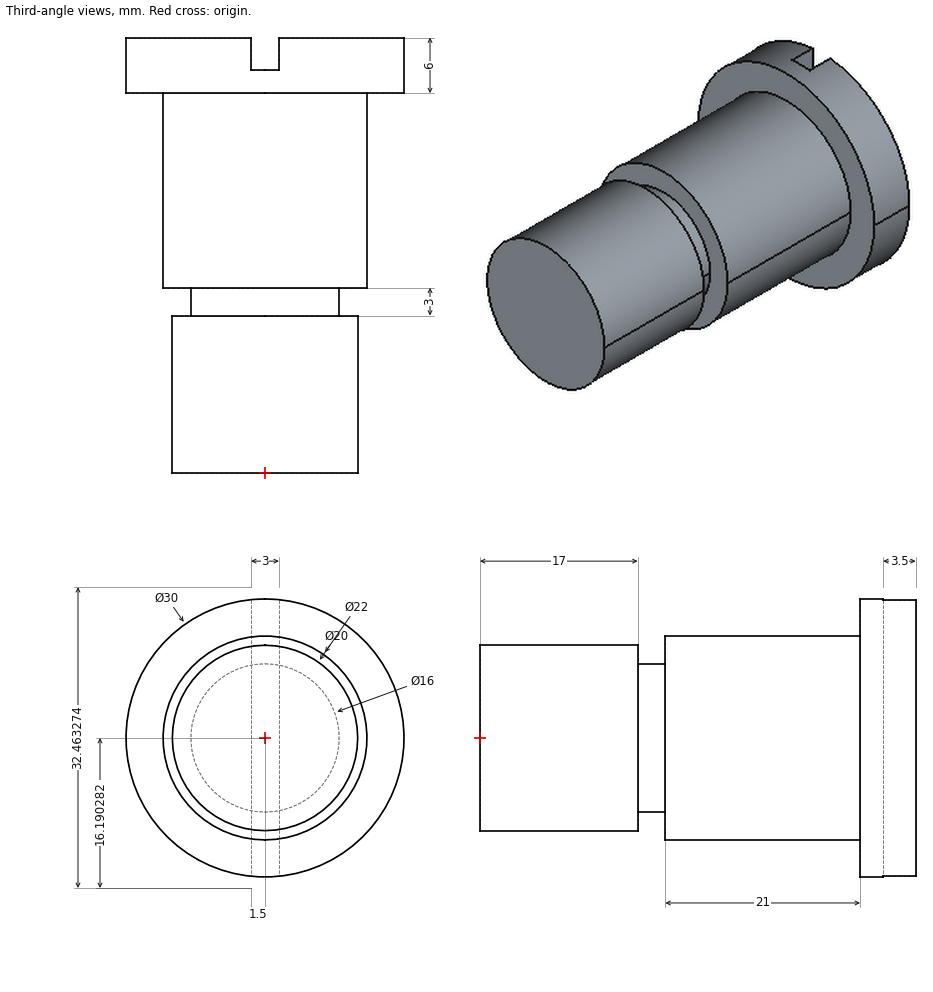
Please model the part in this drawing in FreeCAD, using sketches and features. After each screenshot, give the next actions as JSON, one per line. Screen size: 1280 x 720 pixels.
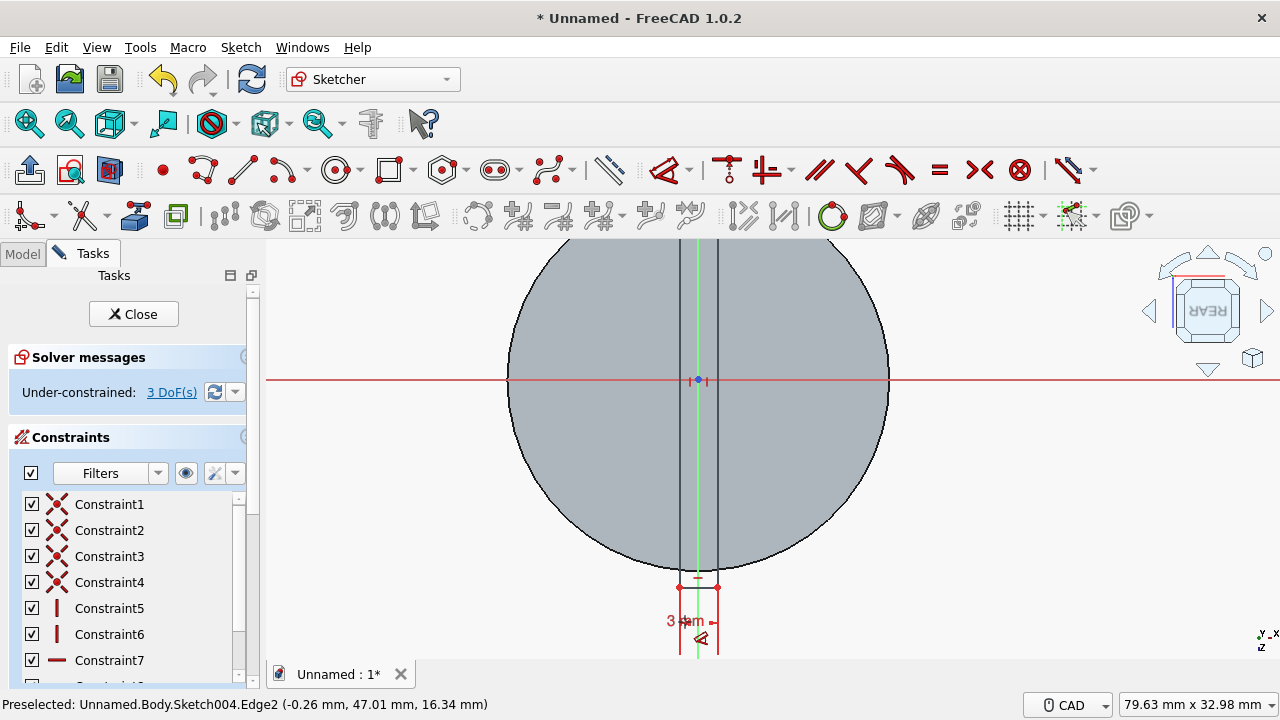
{"action": "scroll", "coordinate": [717, 588], "scroll_direction": "down", "scroll_amount": 2}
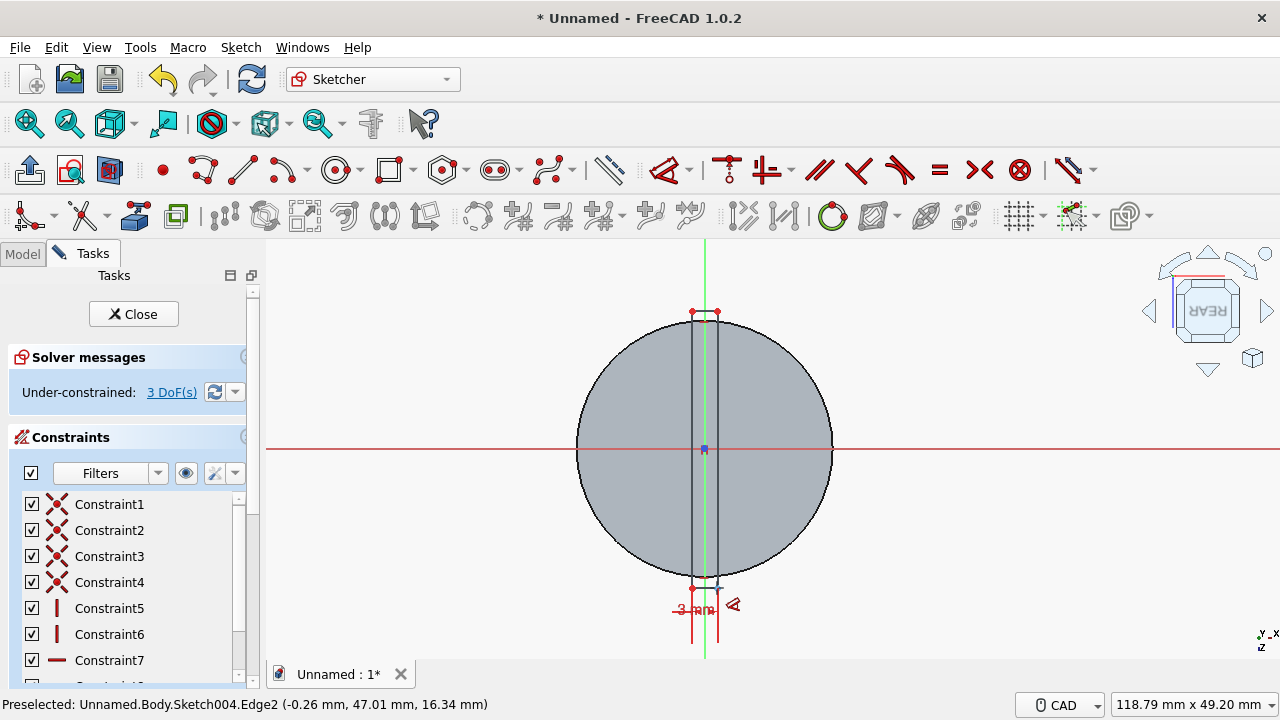
{"action": "scroll", "coordinate": [692, 311], "scroll_direction": "up", "scroll_amount": 6}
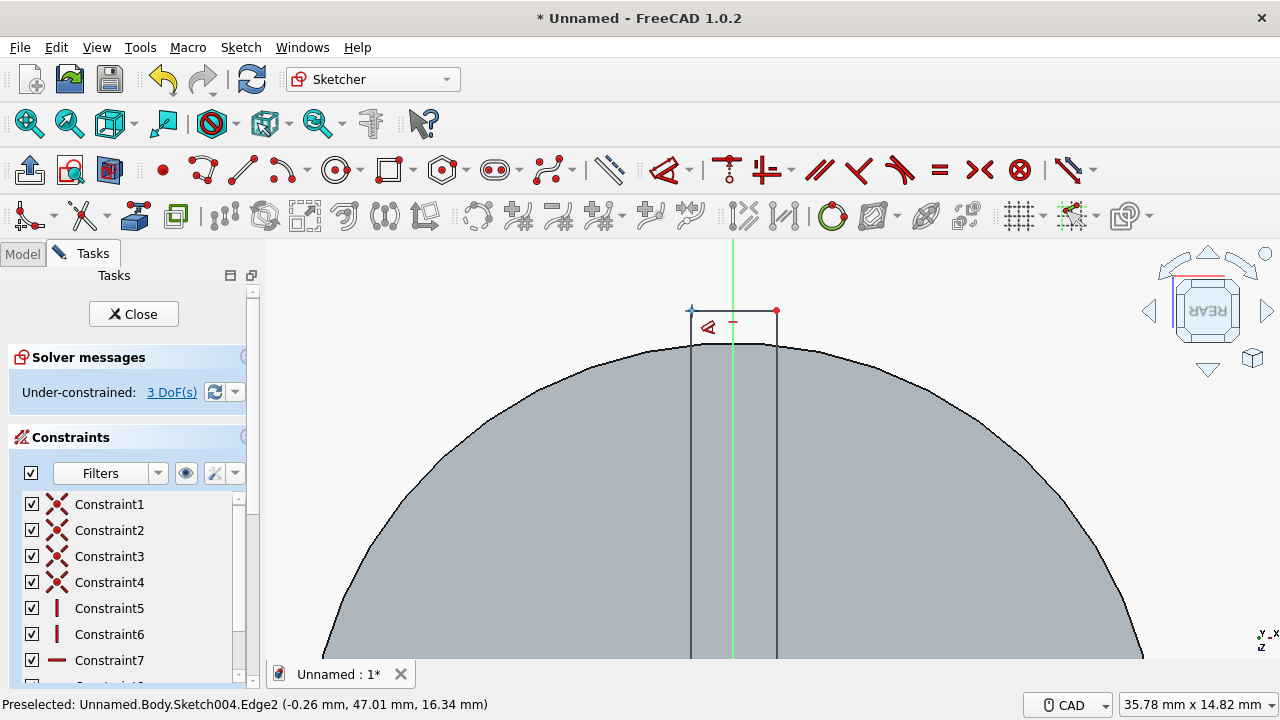
{"action": "left_click", "coordinate": [691, 311]}
{"action": "left_click", "coordinate": [712, 277]}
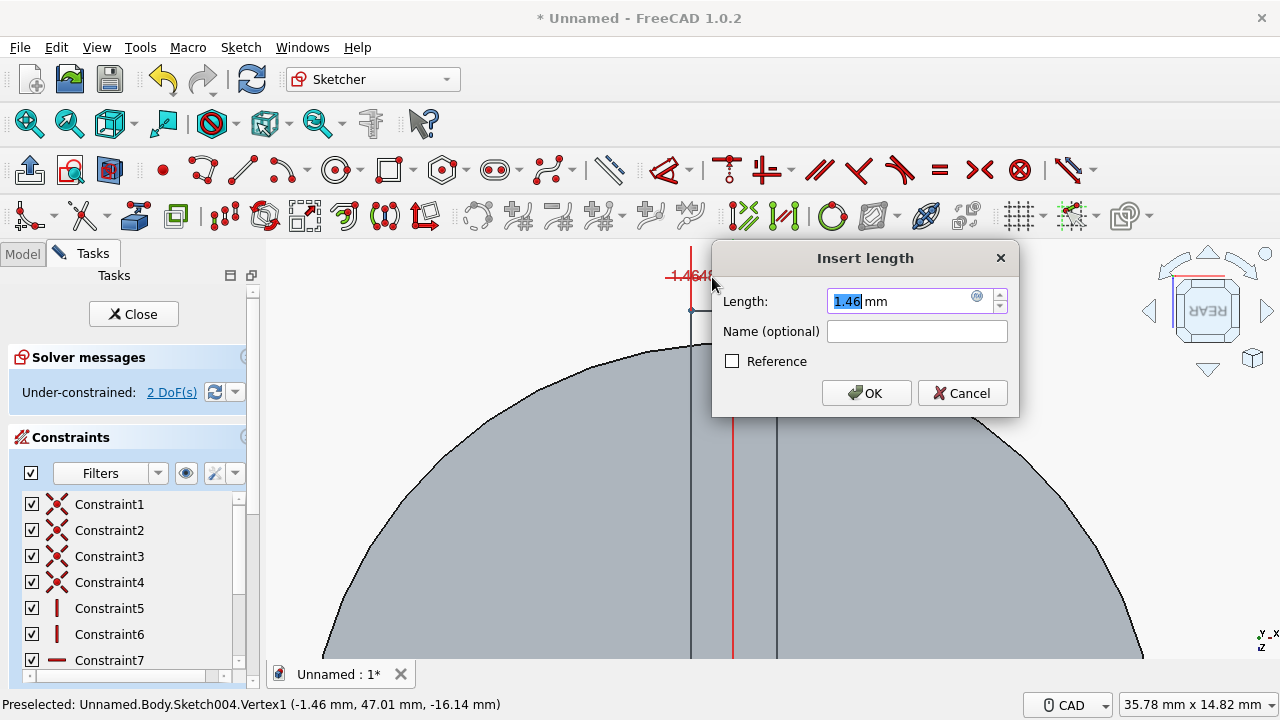
{"action": "type", "text": "1.5"}
{"action": "key", "text": "Return"}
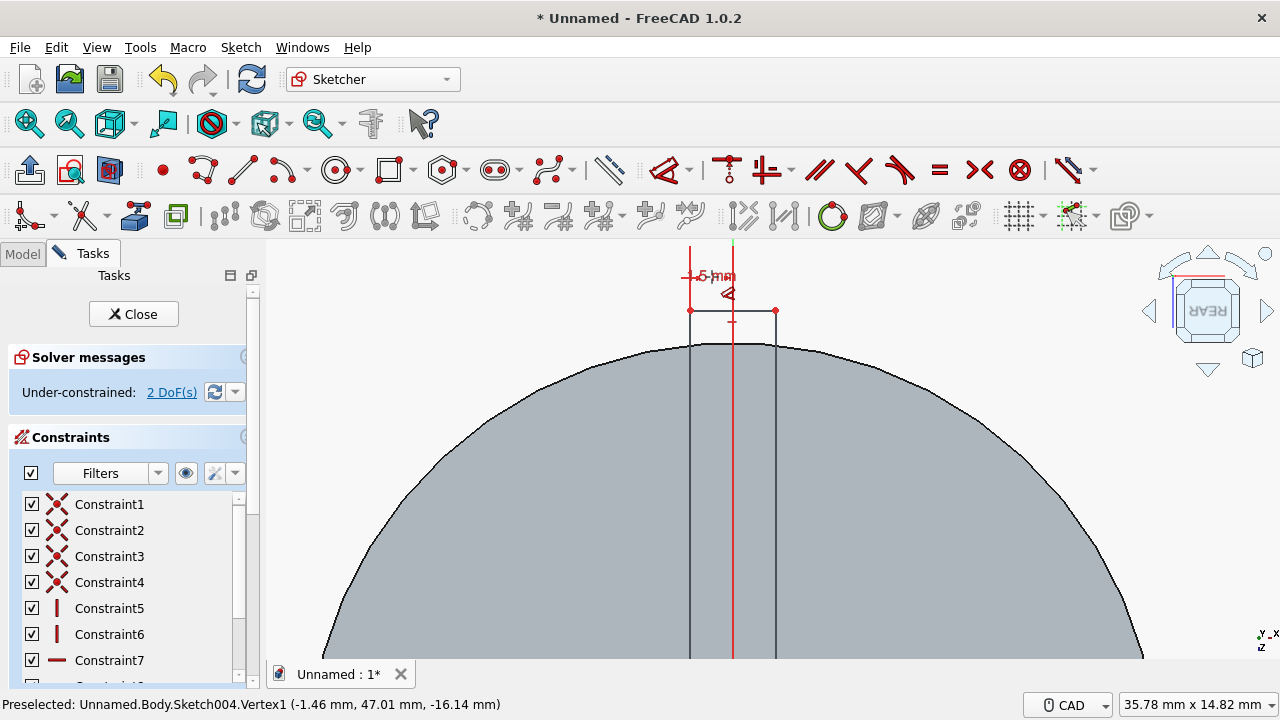
{"action": "left_click", "coordinate": [690, 587]}
{"action": "left_click", "coordinate": [656, 471]}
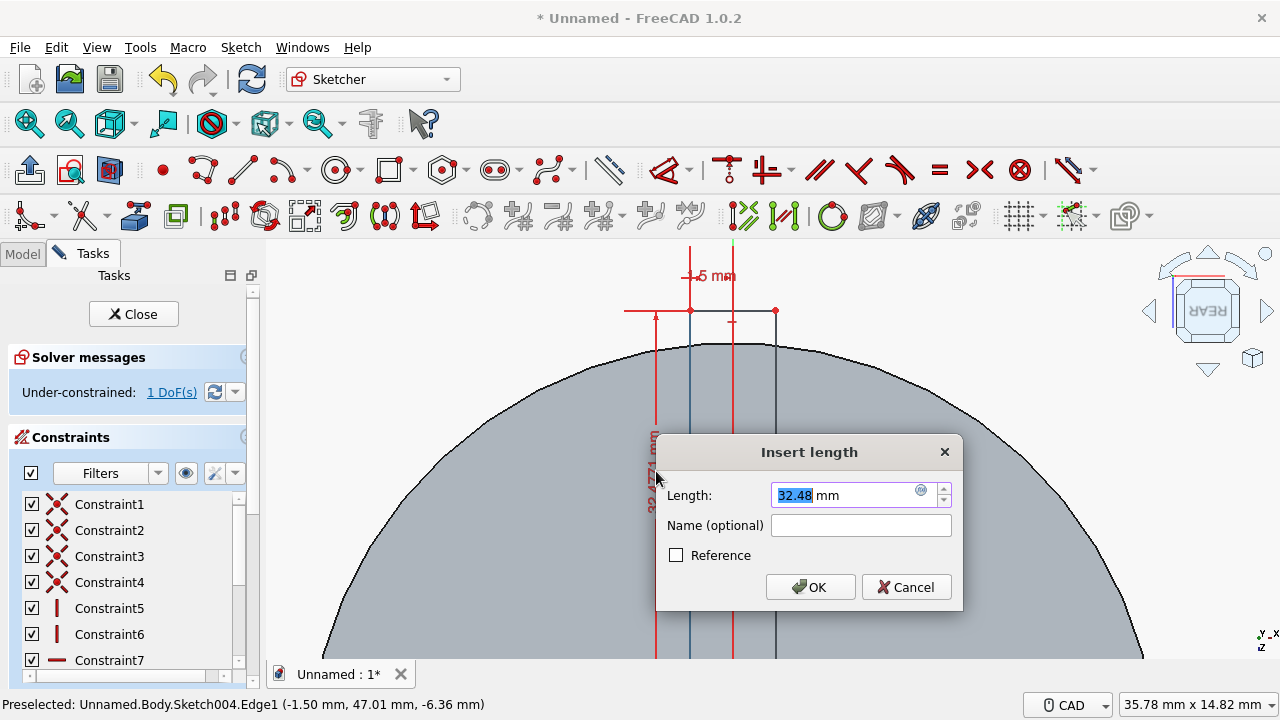
{"action": "type", "text": "32.463274"}
{"action": "key", "text": "Return"}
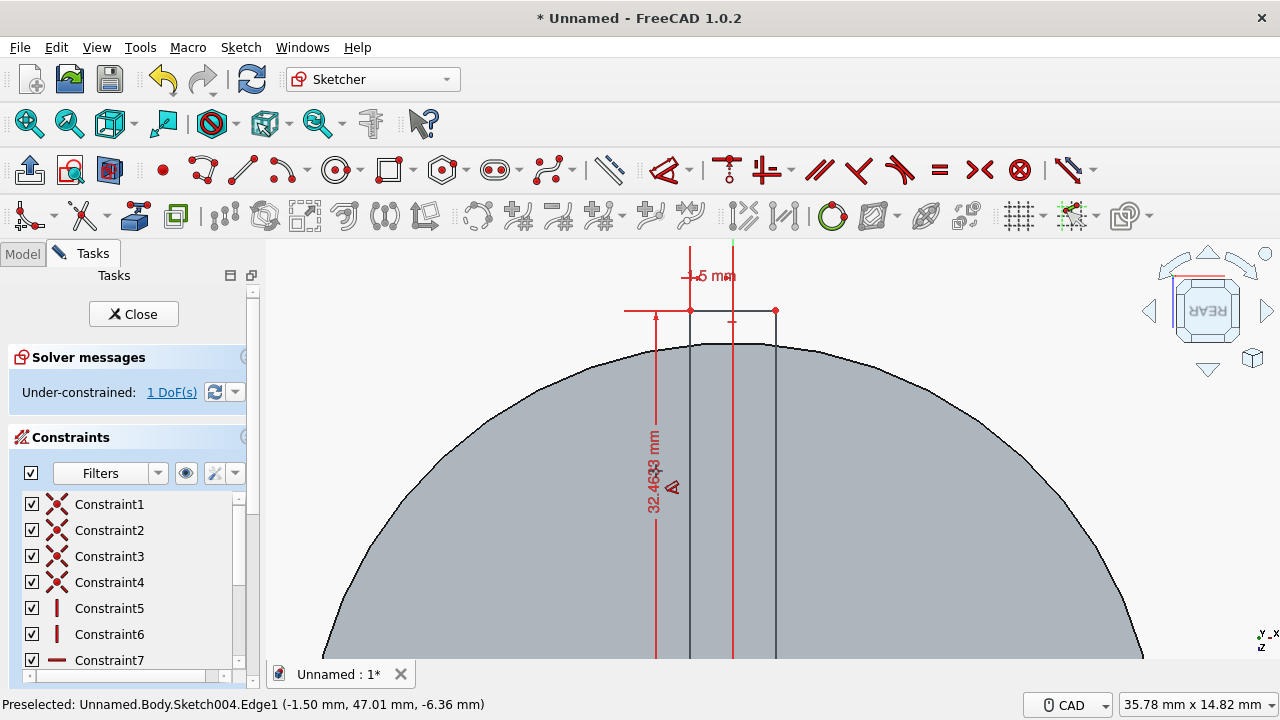
{"action": "left_click", "coordinate": [690, 311]}
{"action": "left_click", "coordinate": [656, 397]}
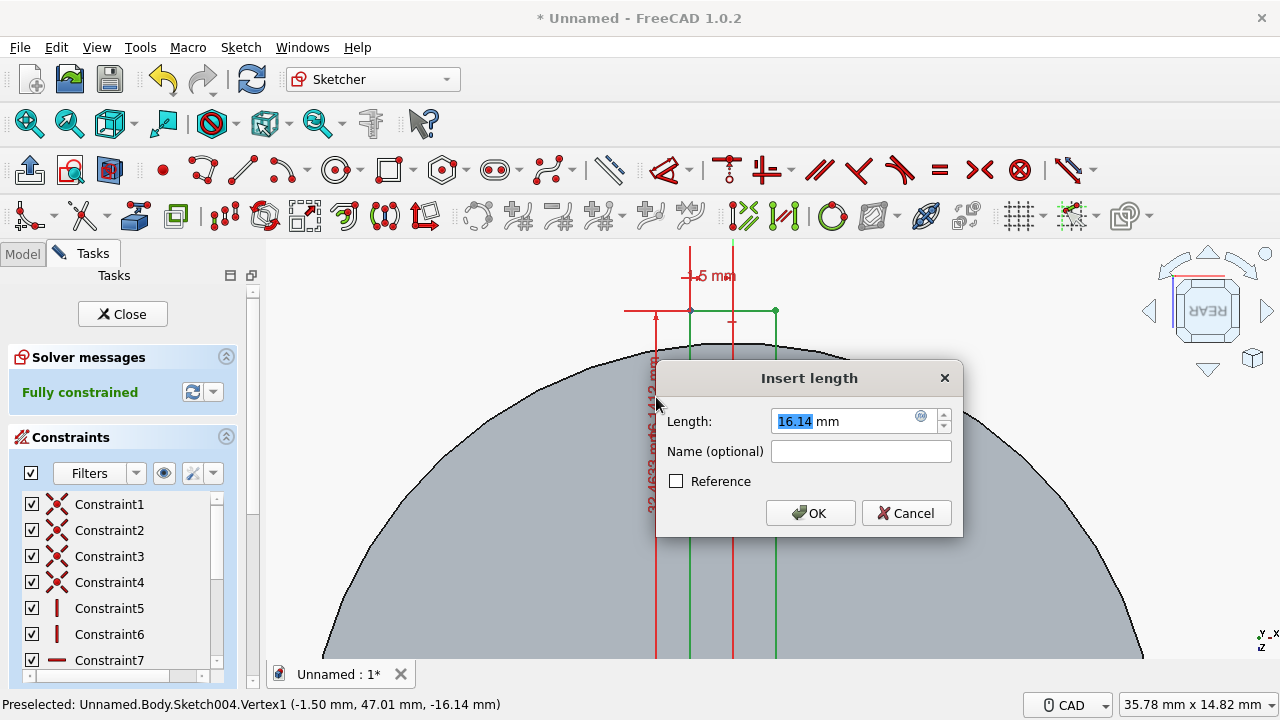
{"action": "type", "text": "16.190282"}
{"action": "key", "text": "Return"}
{"action": "key", "text": "Escape"}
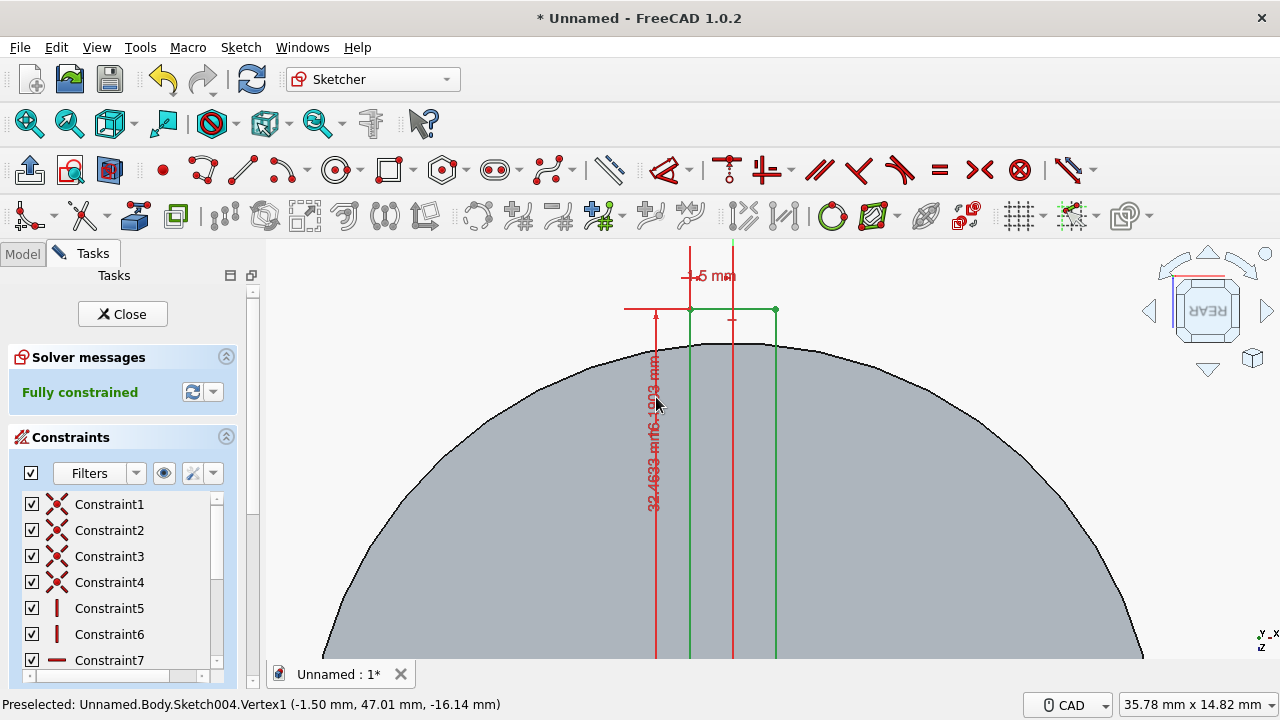
{"action": "left_click", "coordinate": [123, 314]}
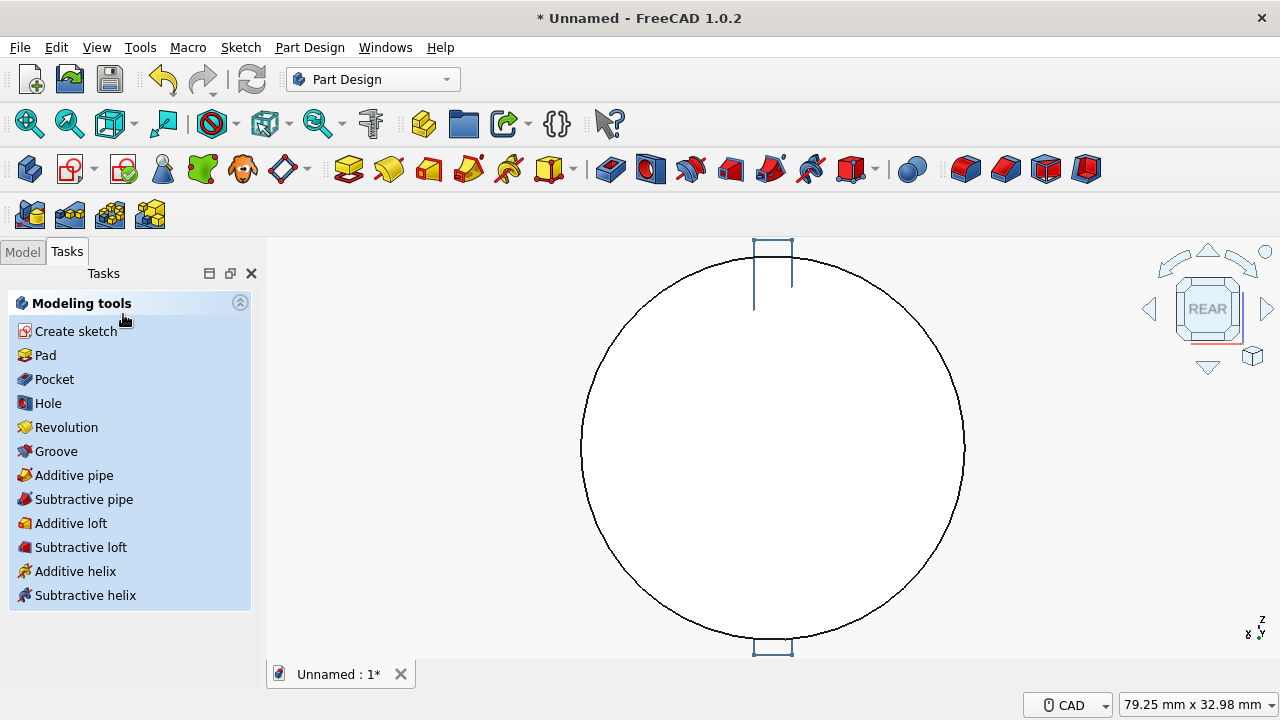
{"action": "left_click", "coordinate": [612, 170]}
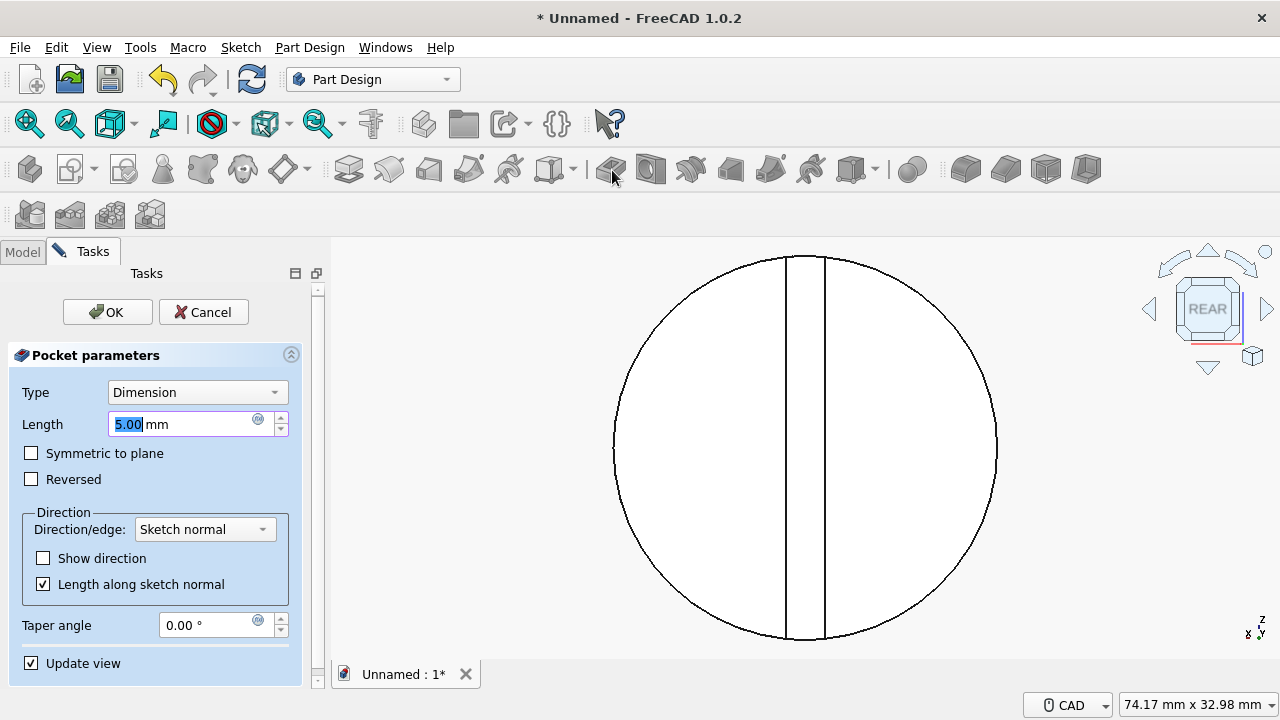
{"action": "type", "text": "3.5"}
{"action": "key", "text": "Tab"}